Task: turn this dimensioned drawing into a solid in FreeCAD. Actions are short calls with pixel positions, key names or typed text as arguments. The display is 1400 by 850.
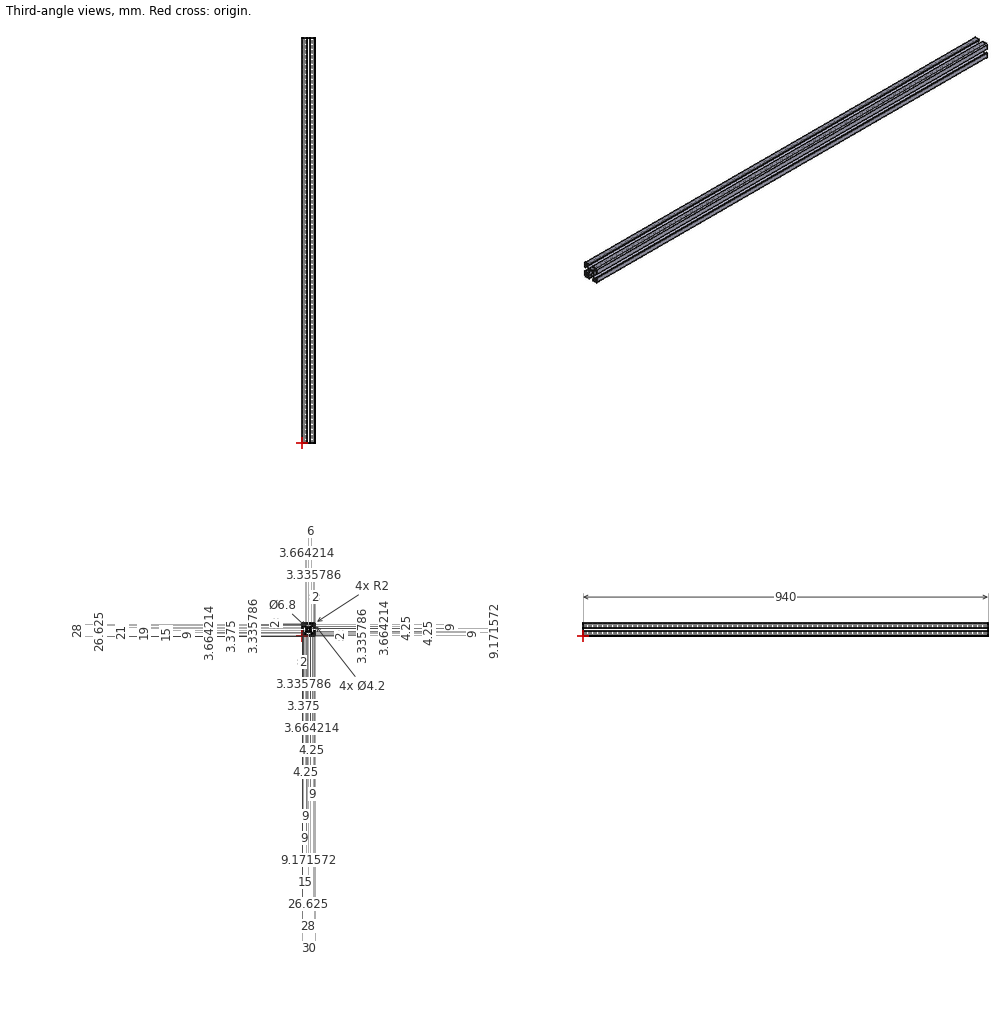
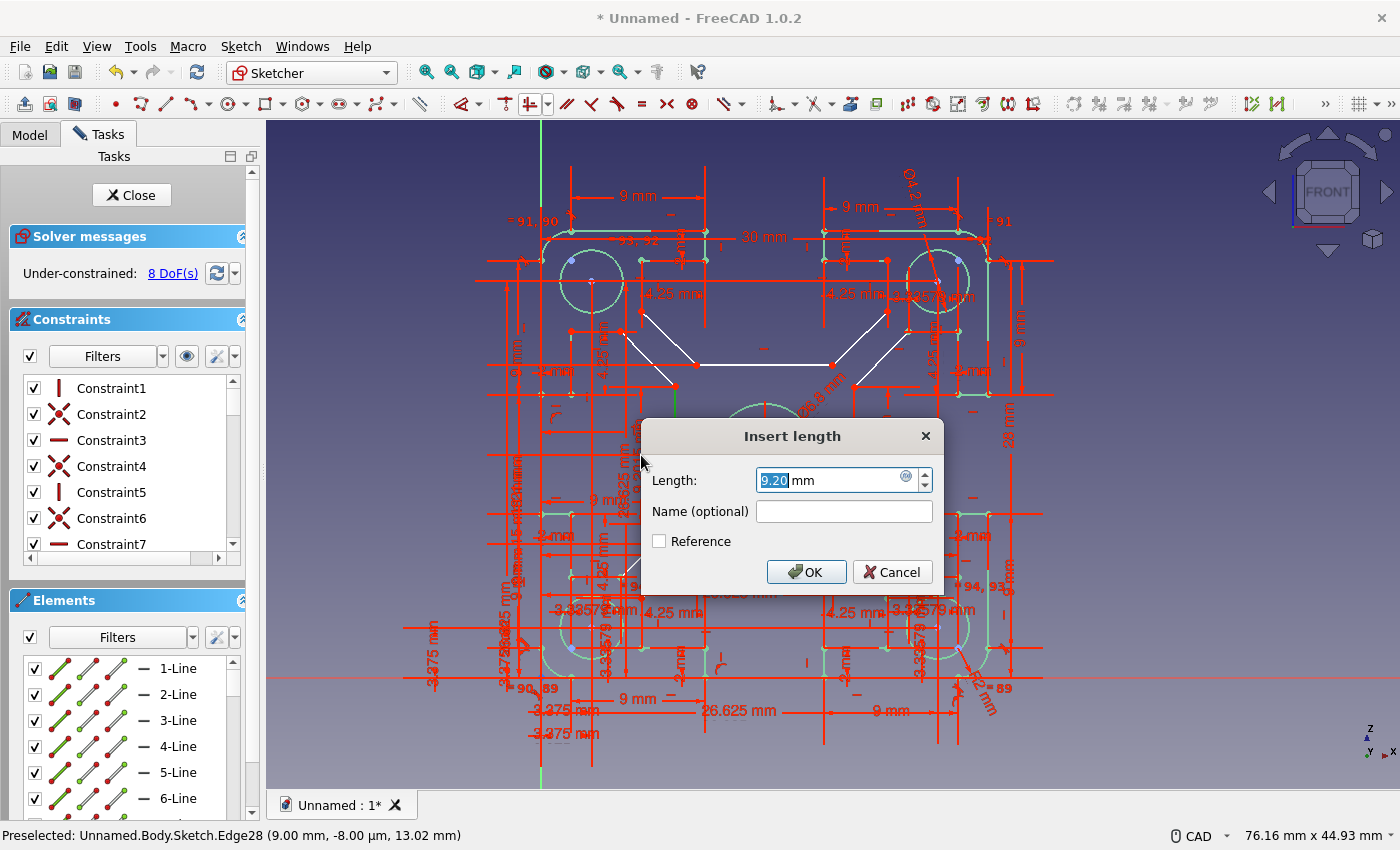
text(9.171572)
key(Return)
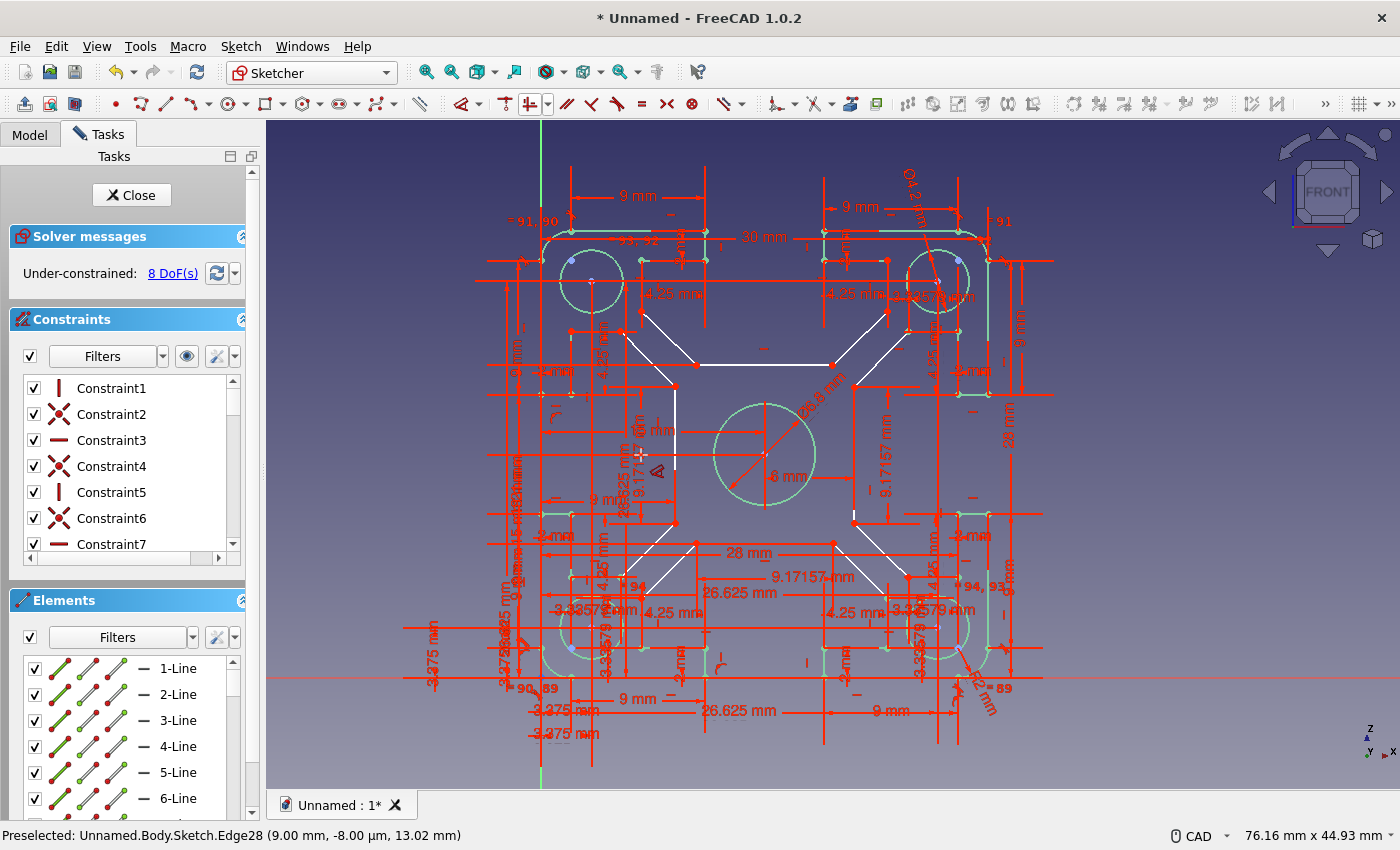
click(606, 332)
click(596, 298)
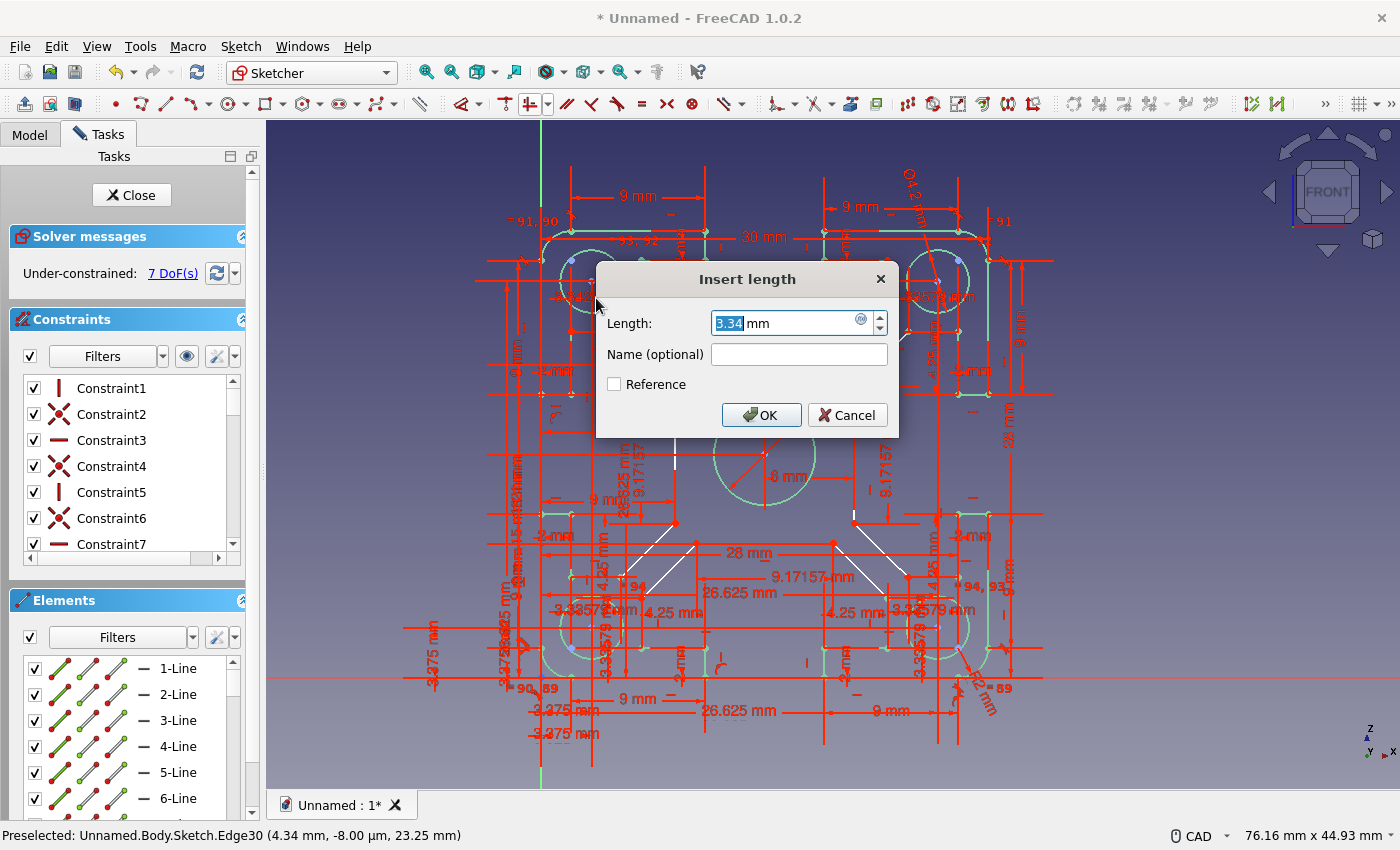
text(3.335786)
key(Return)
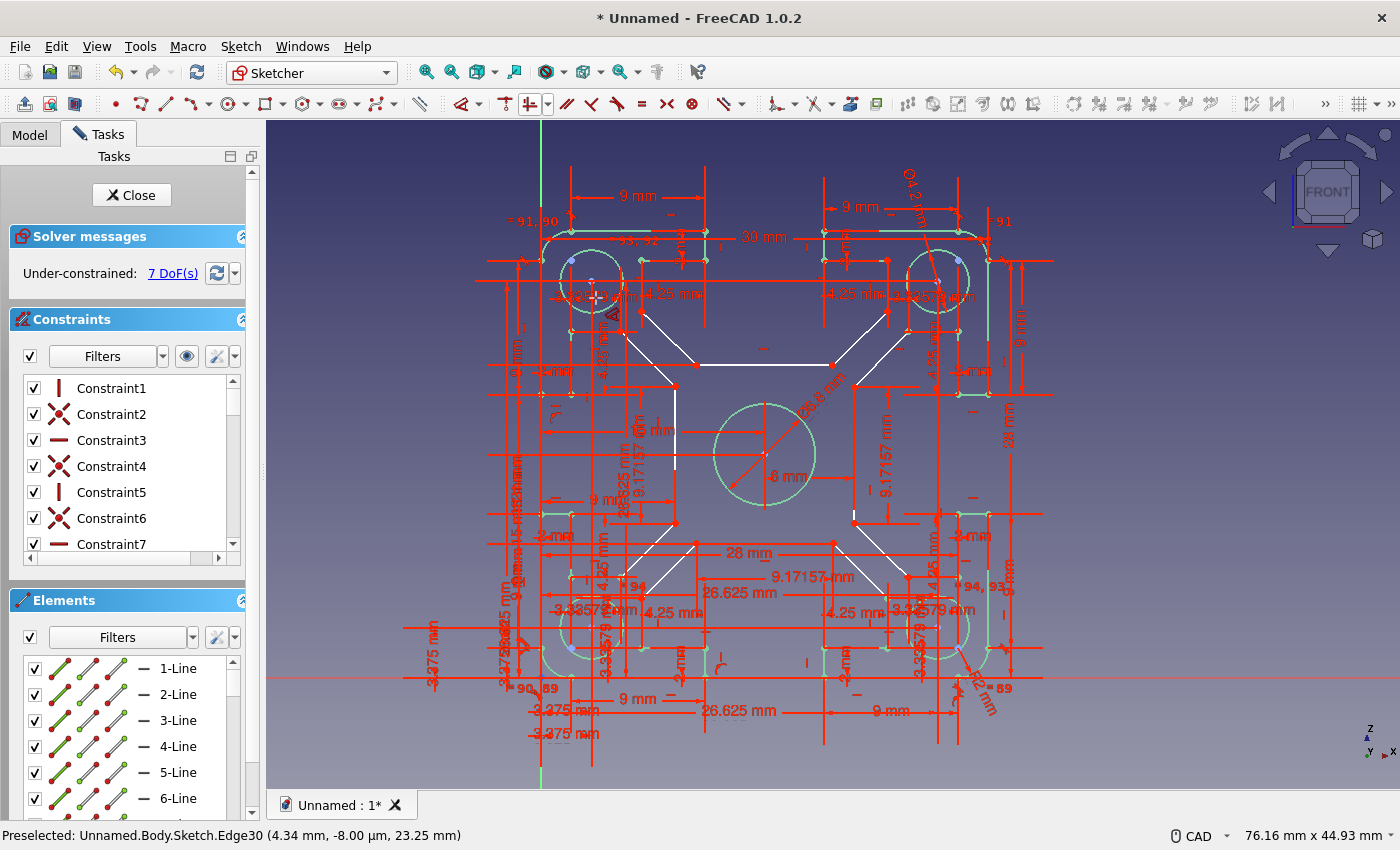
click(642, 276)
click(608, 275)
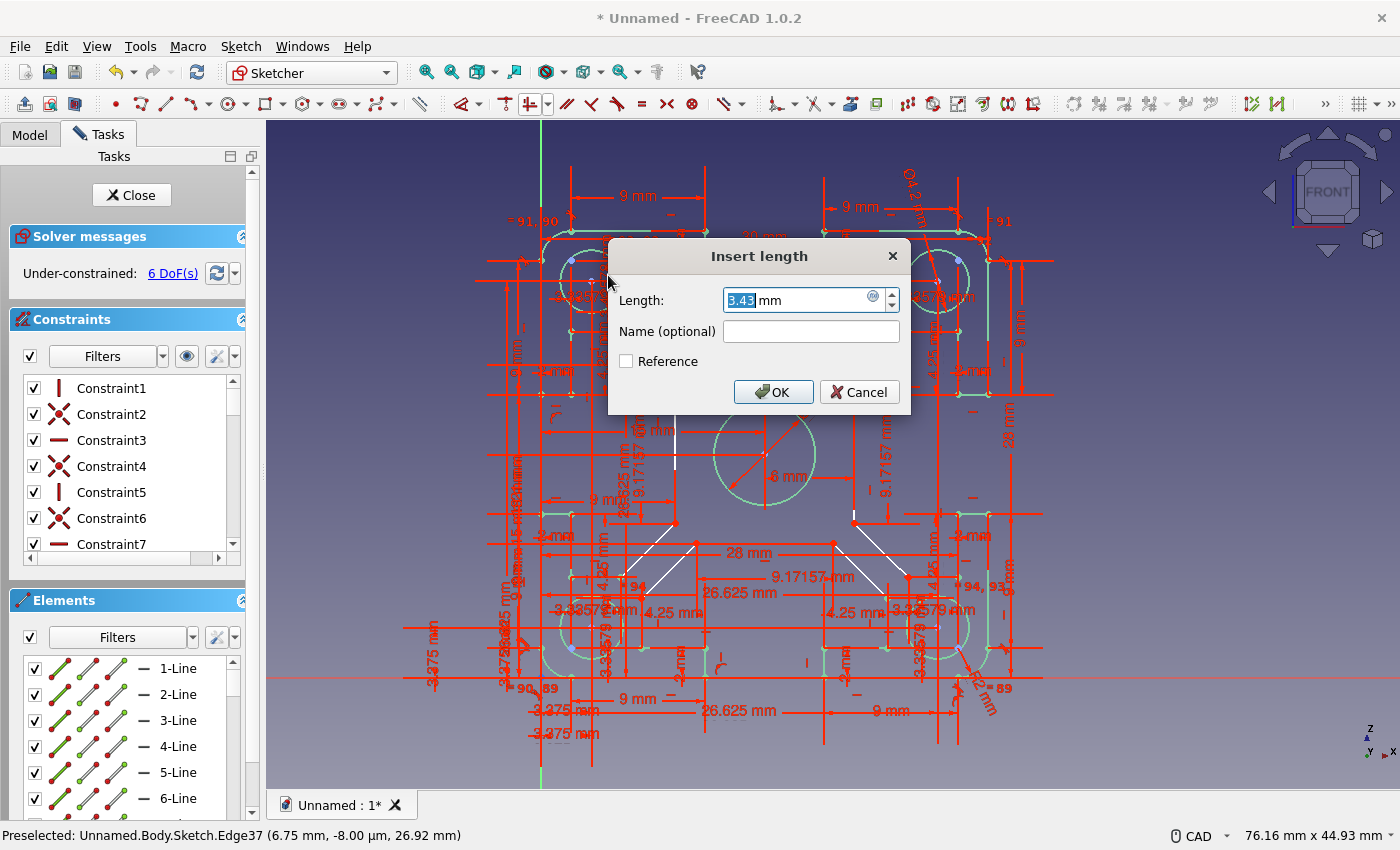
text(3.335786)
key(Return)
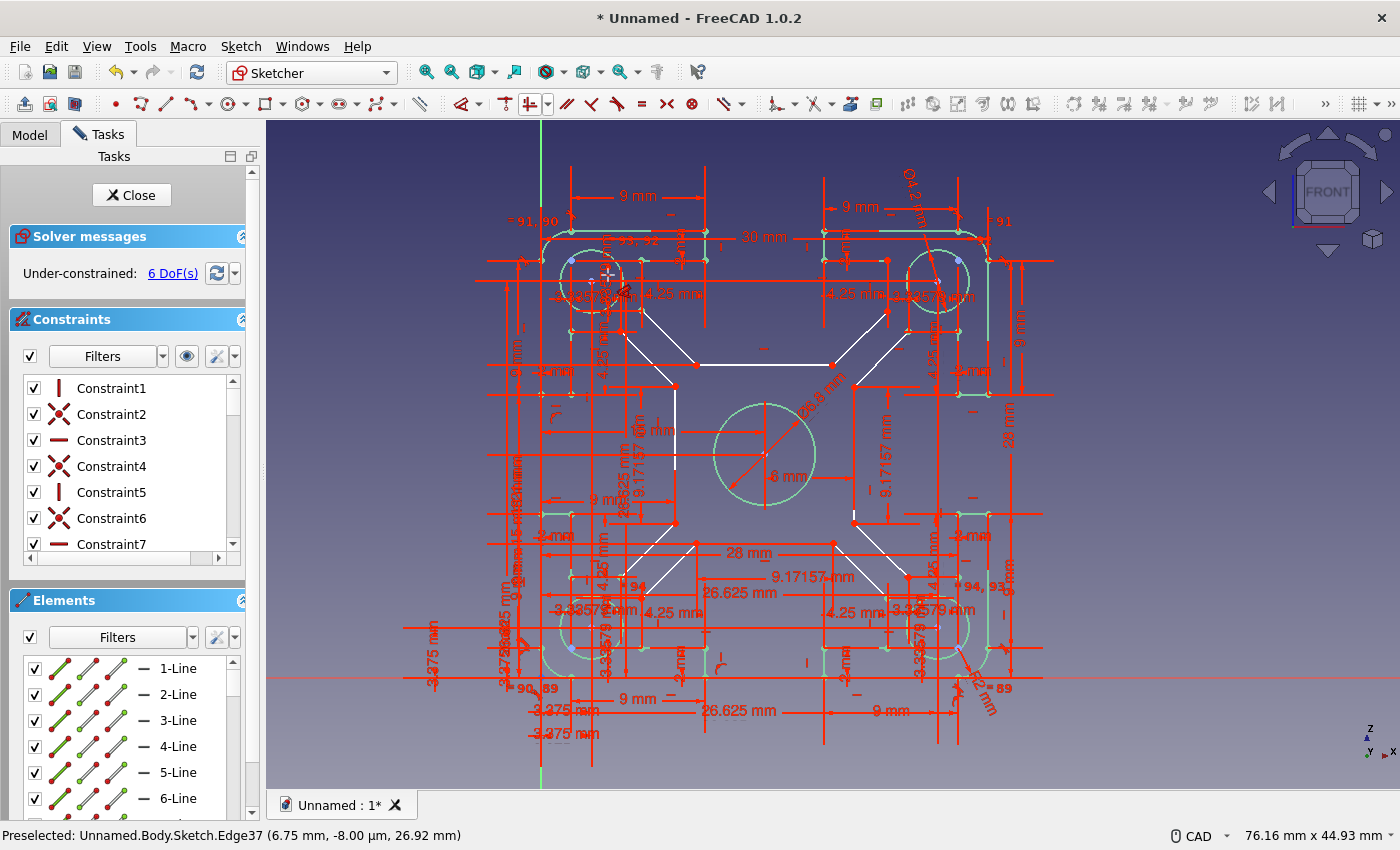
click(738, 365)
click(765, 331)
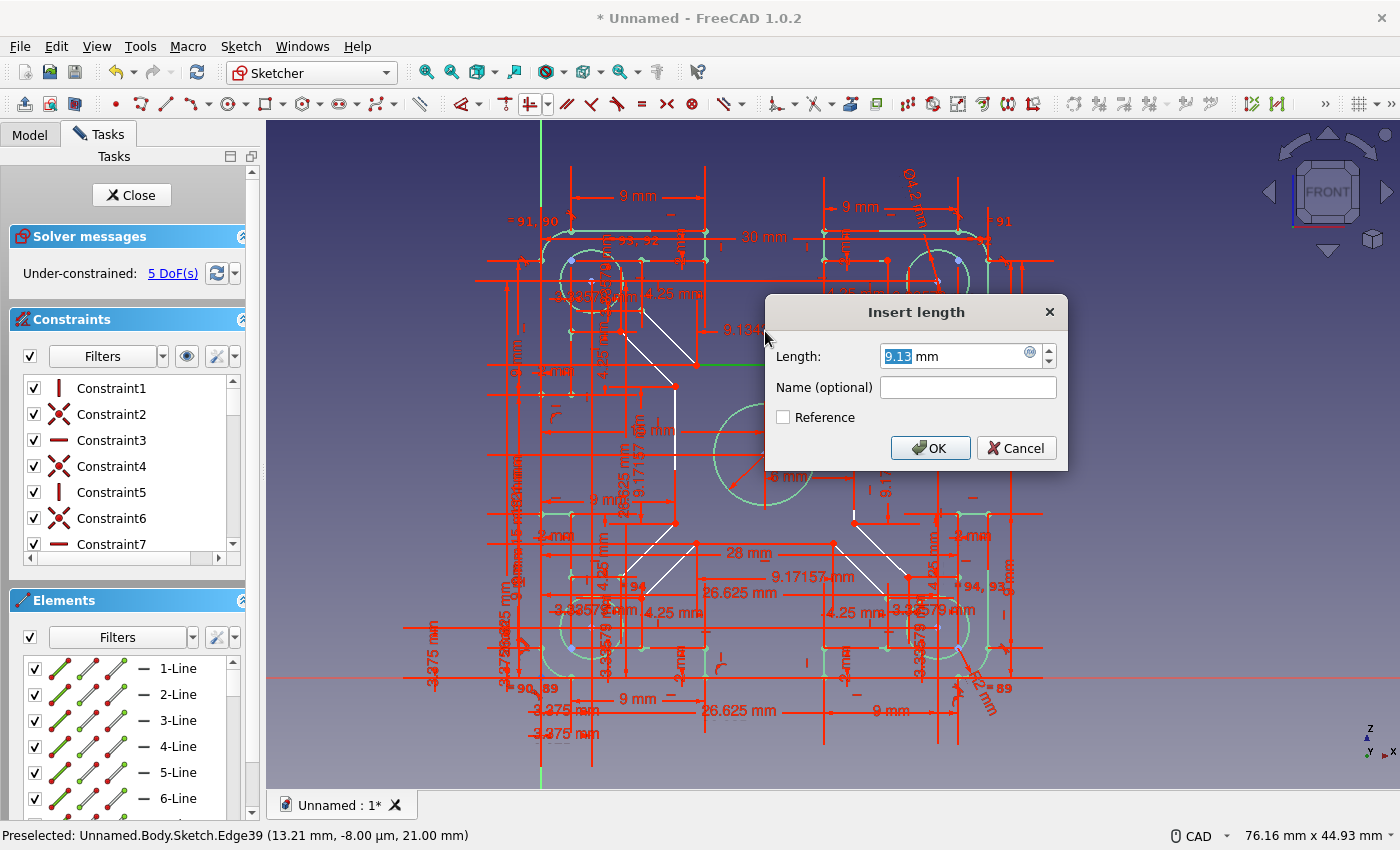
text(9.171572)
key(Return)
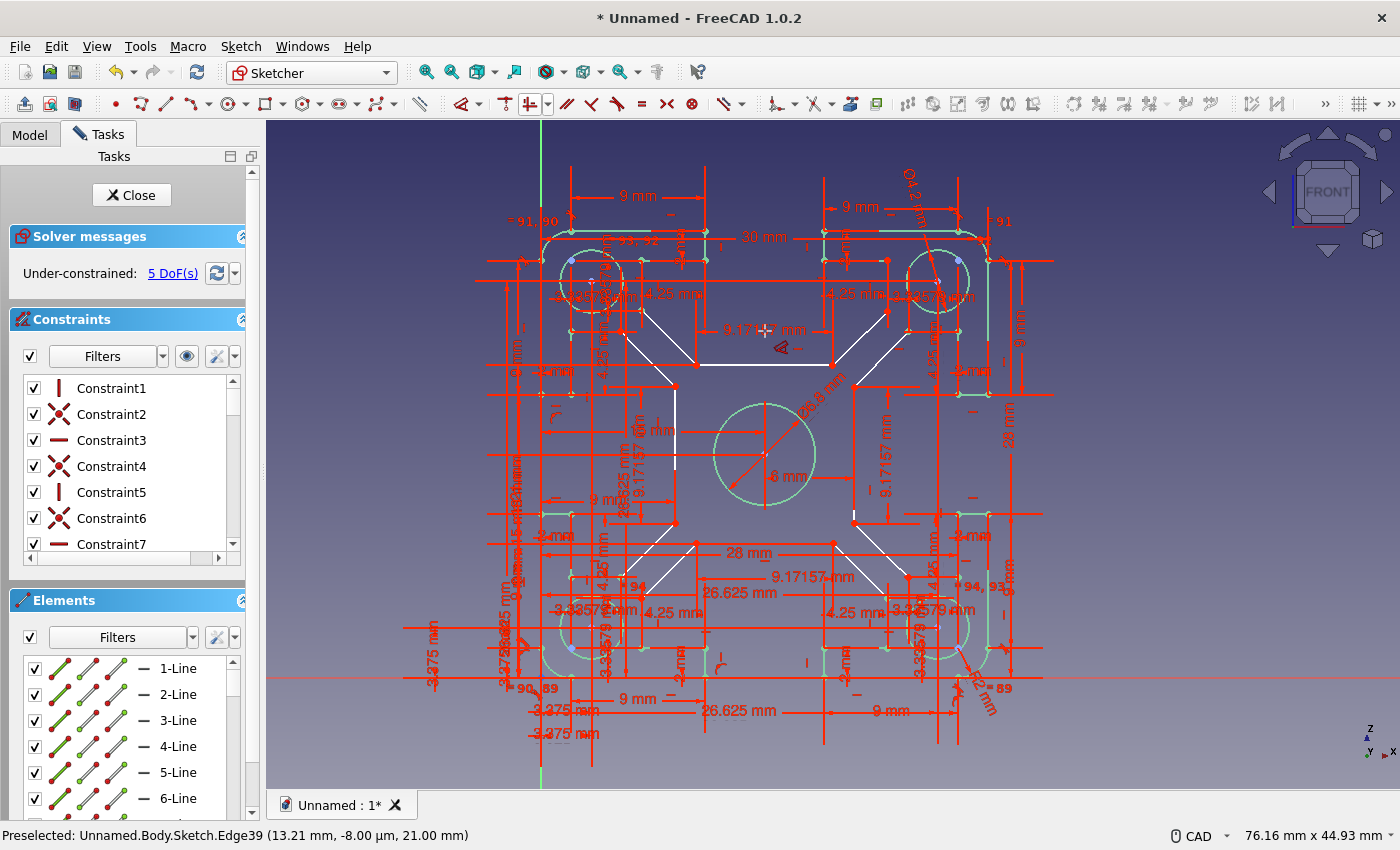
click(888, 297)
click(922, 275)